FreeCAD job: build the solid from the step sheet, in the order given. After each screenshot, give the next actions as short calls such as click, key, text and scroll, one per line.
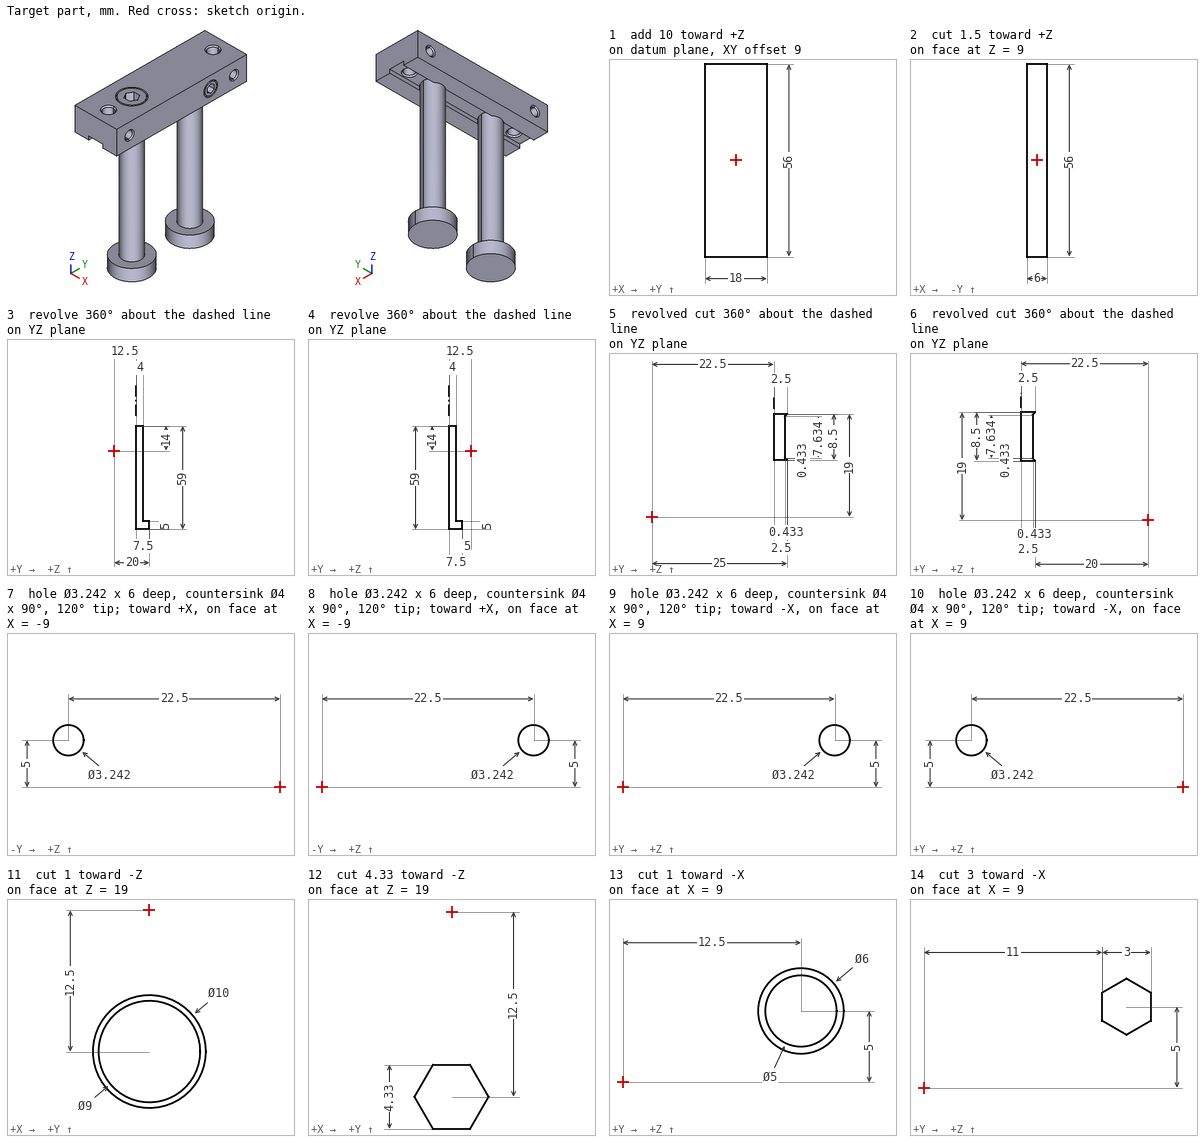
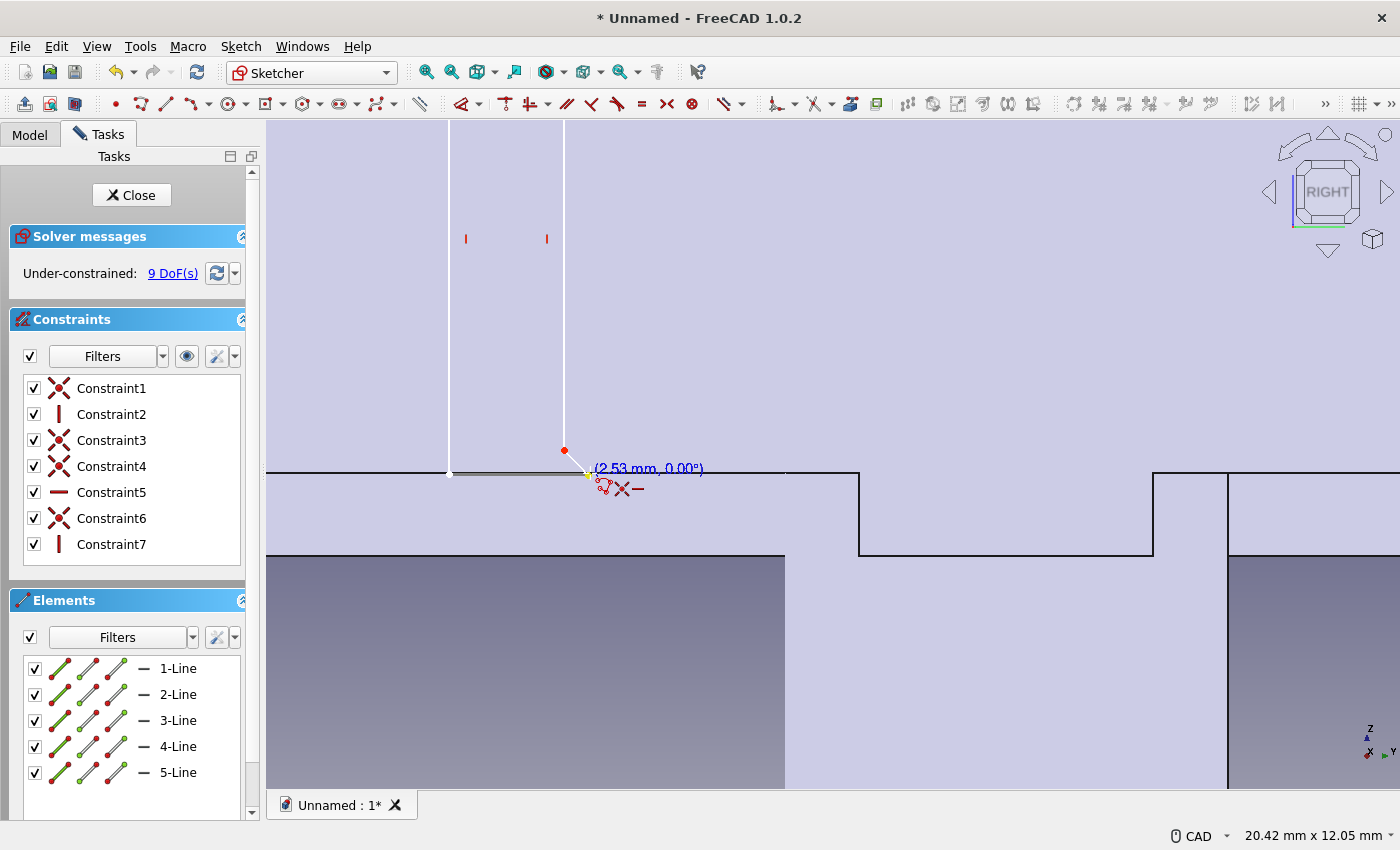
click(588, 476)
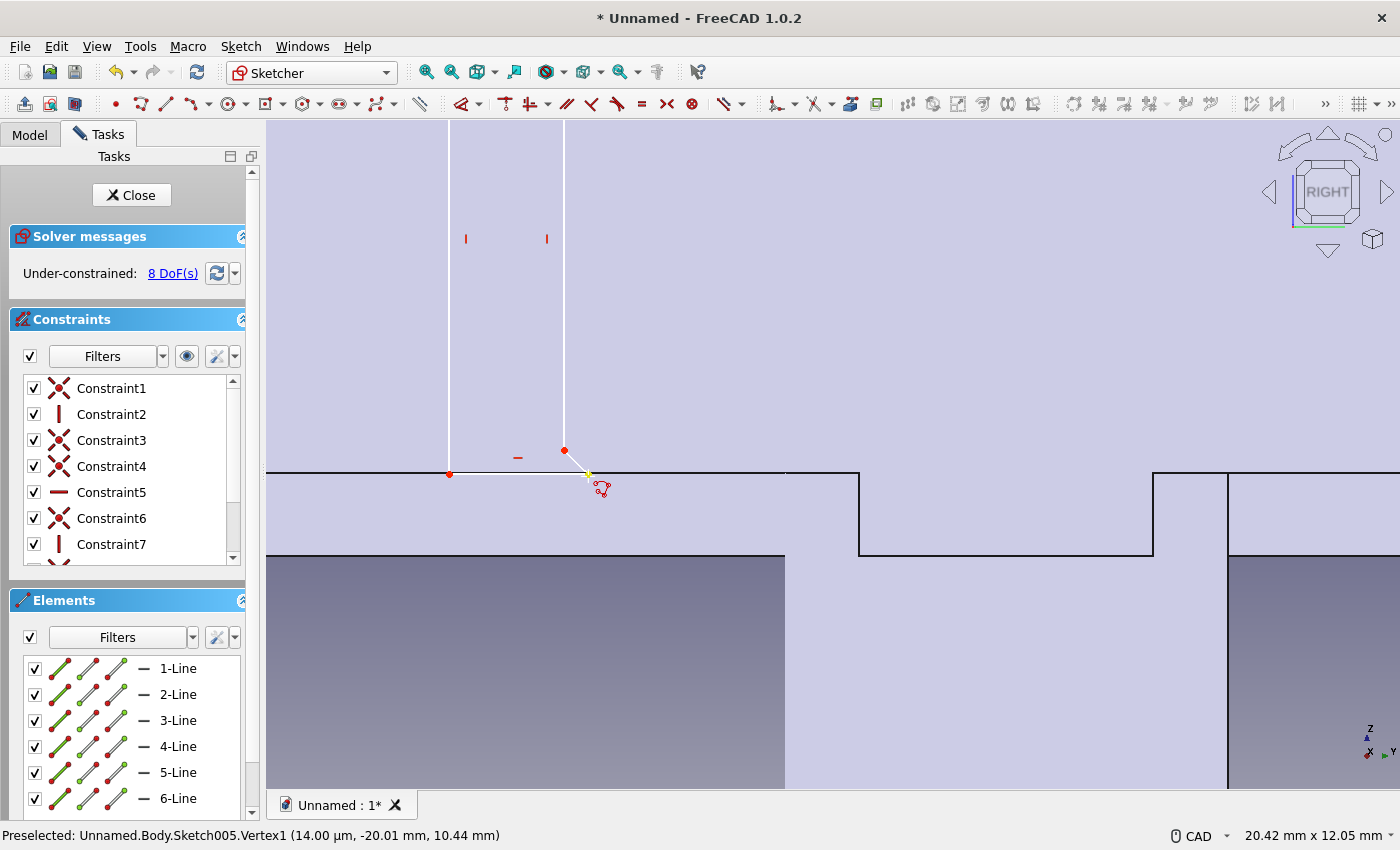
click(166, 104)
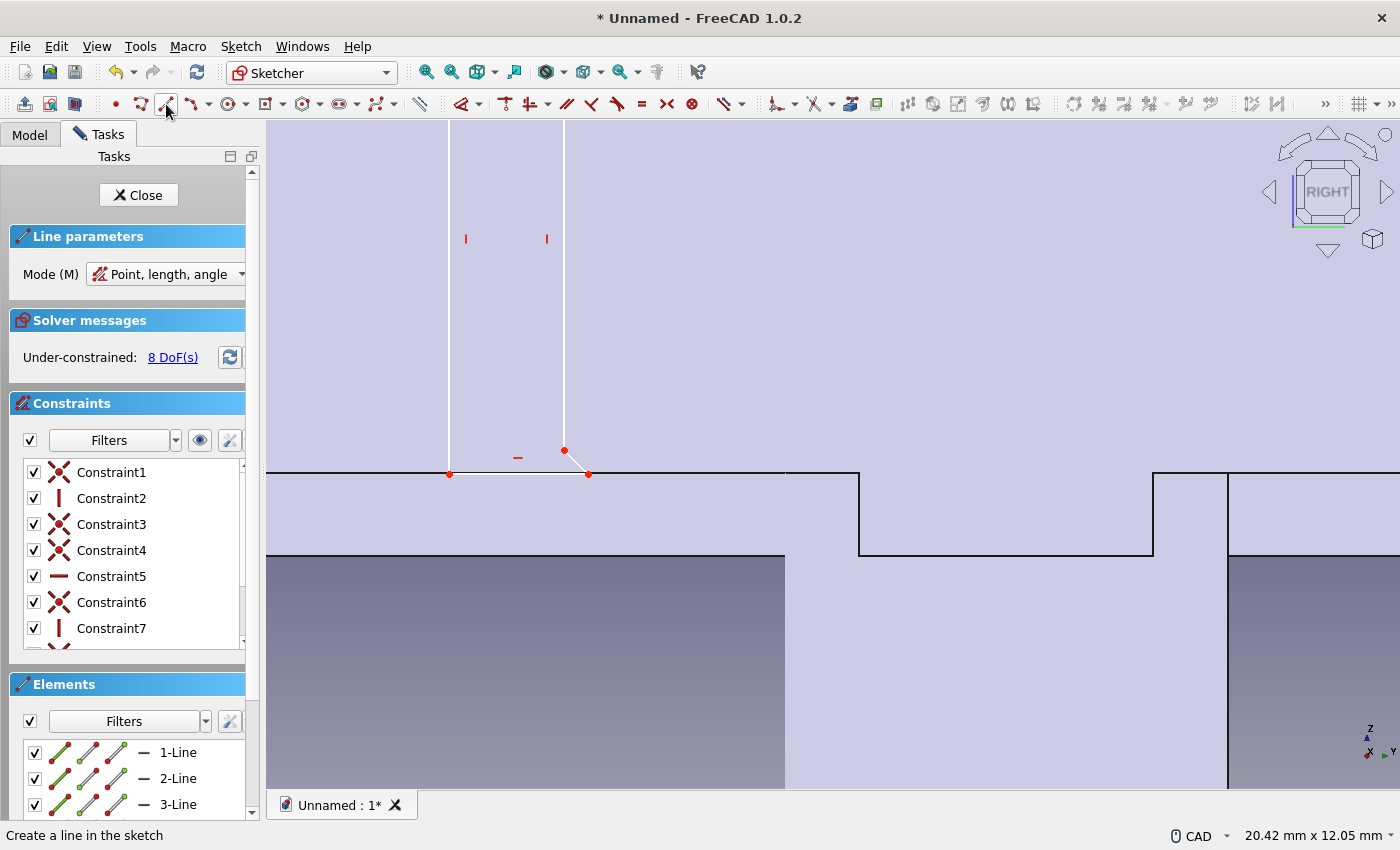
scroll(584, 467, down, 5)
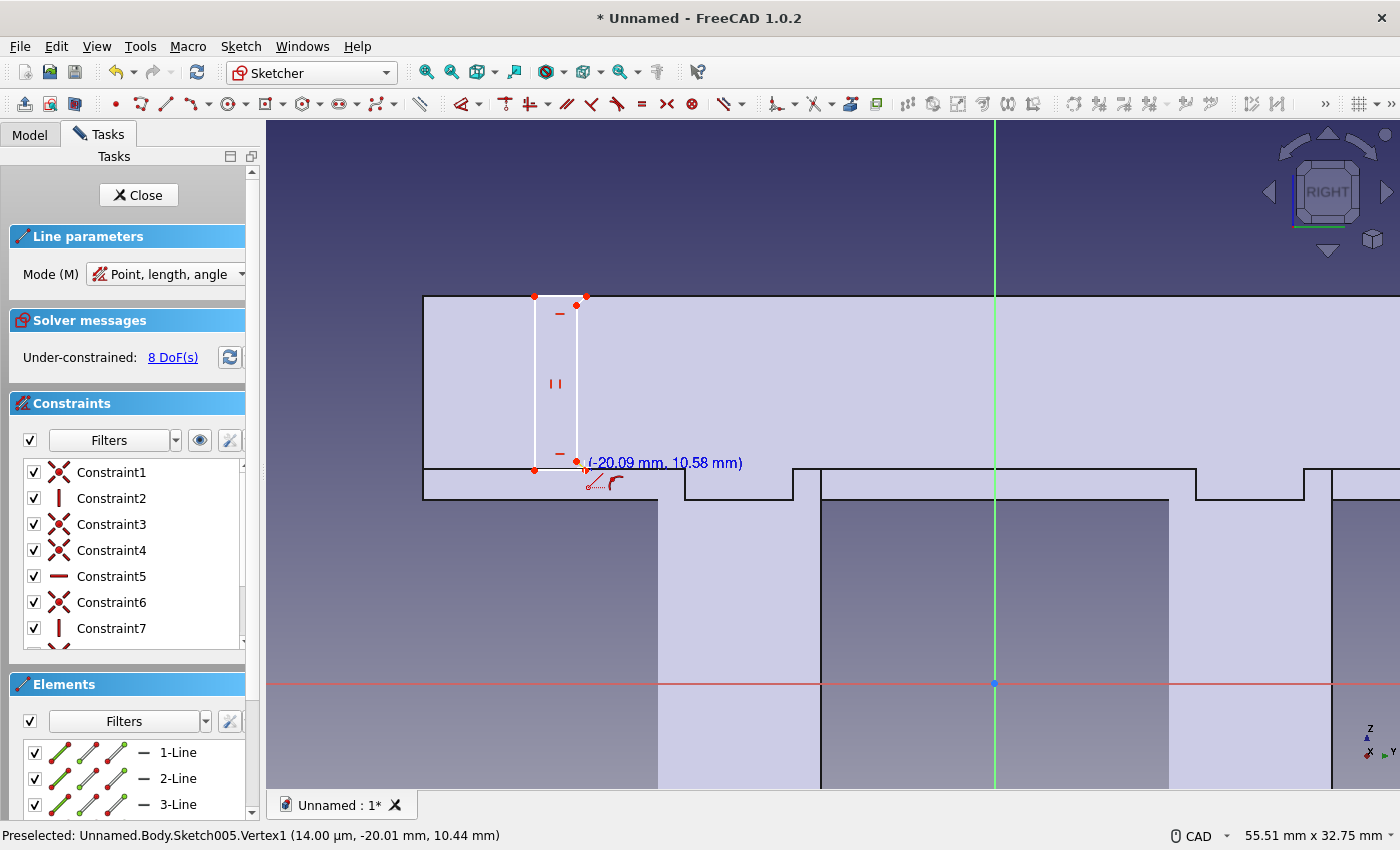
click(535, 278)
click(535, 226)
key(Escape)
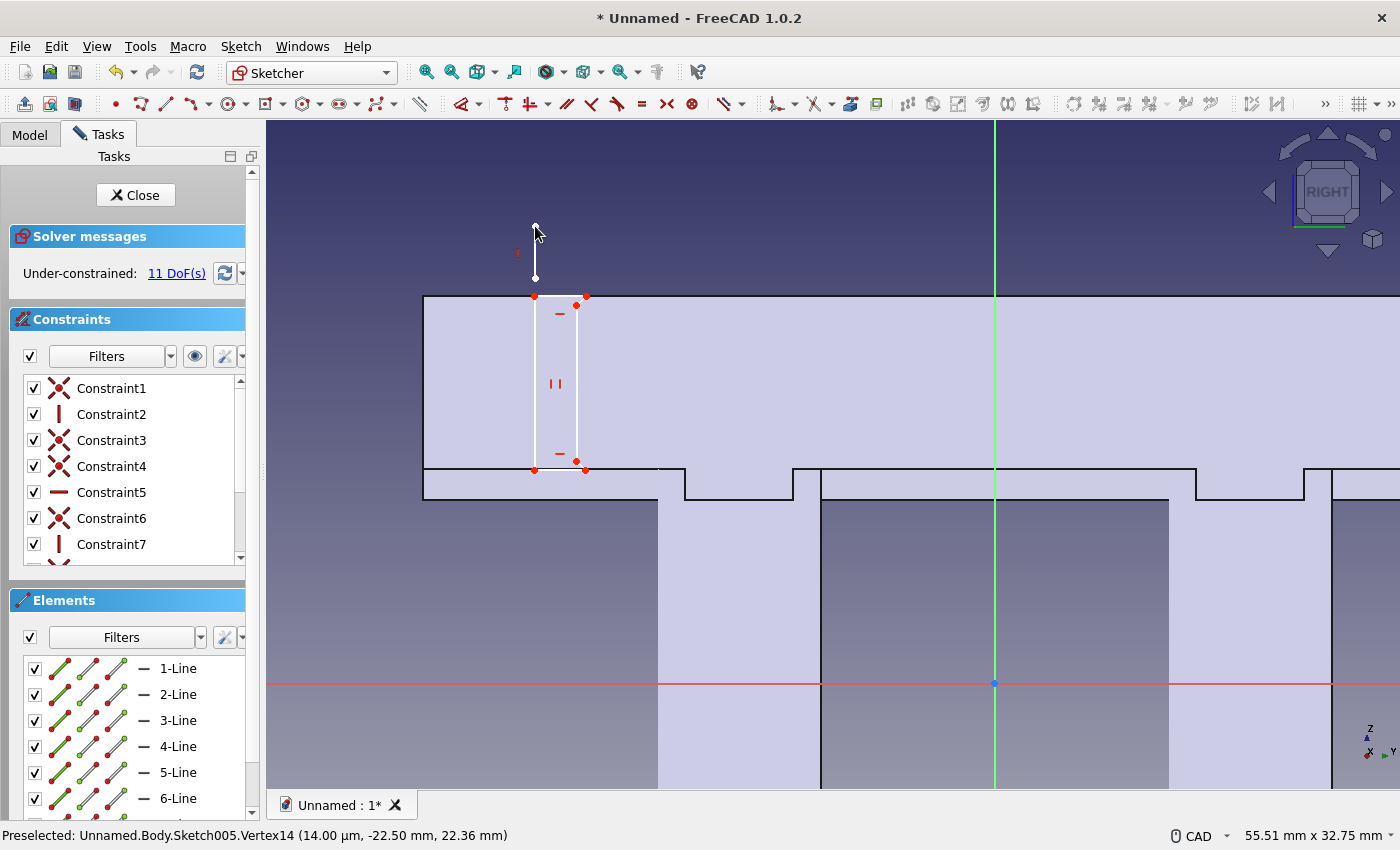
click(535, 263)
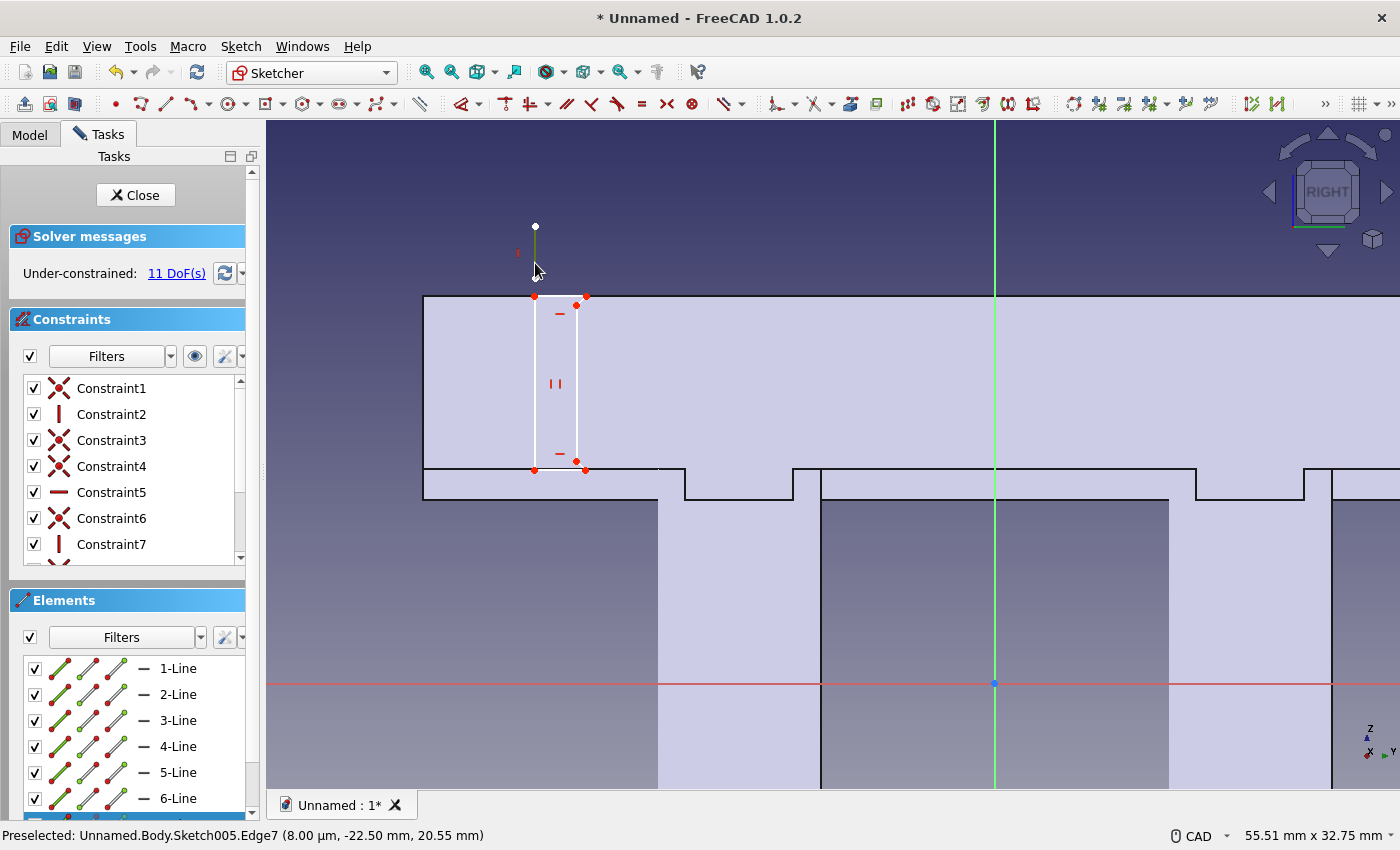
click(420, 104)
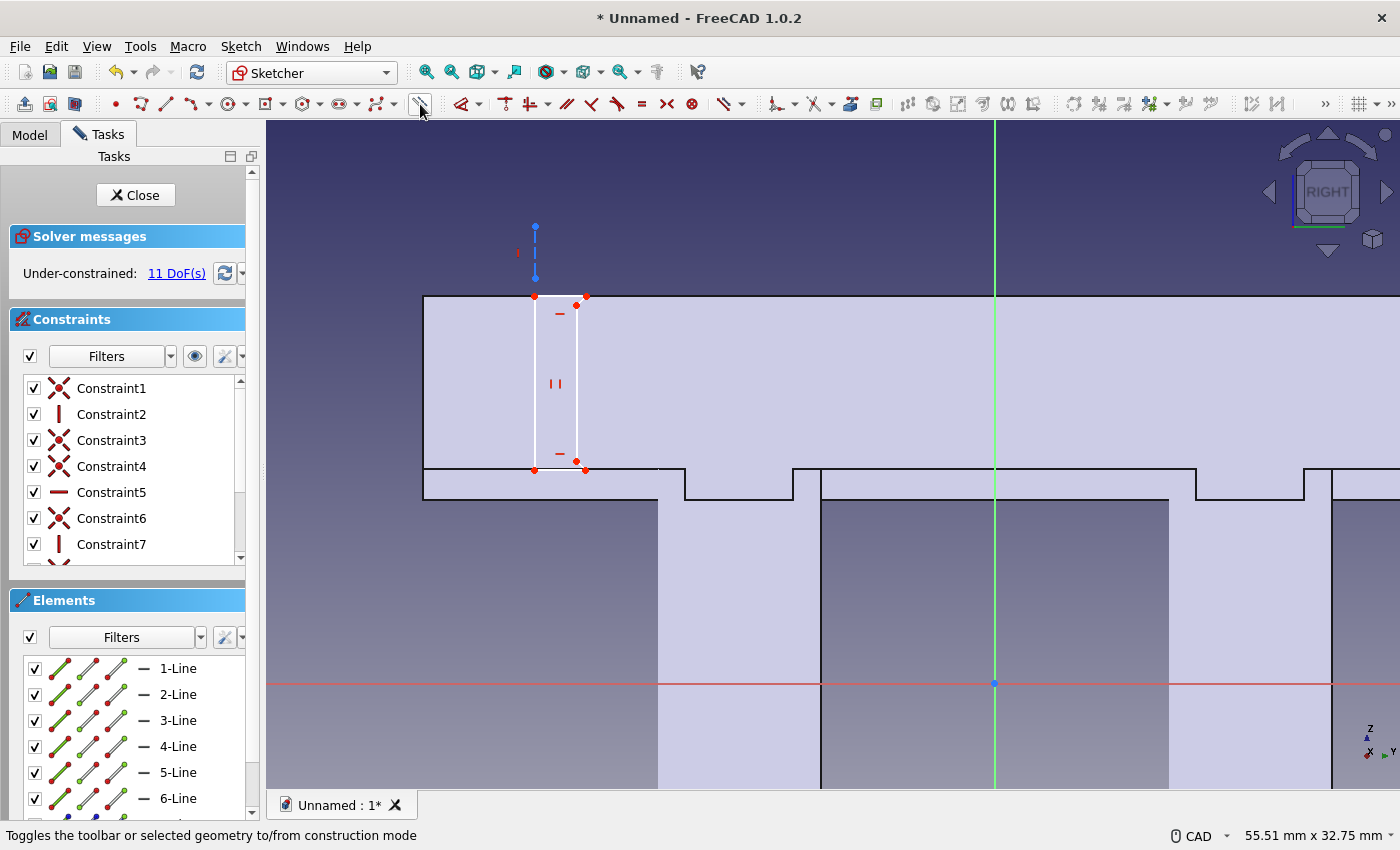
click(460, 104)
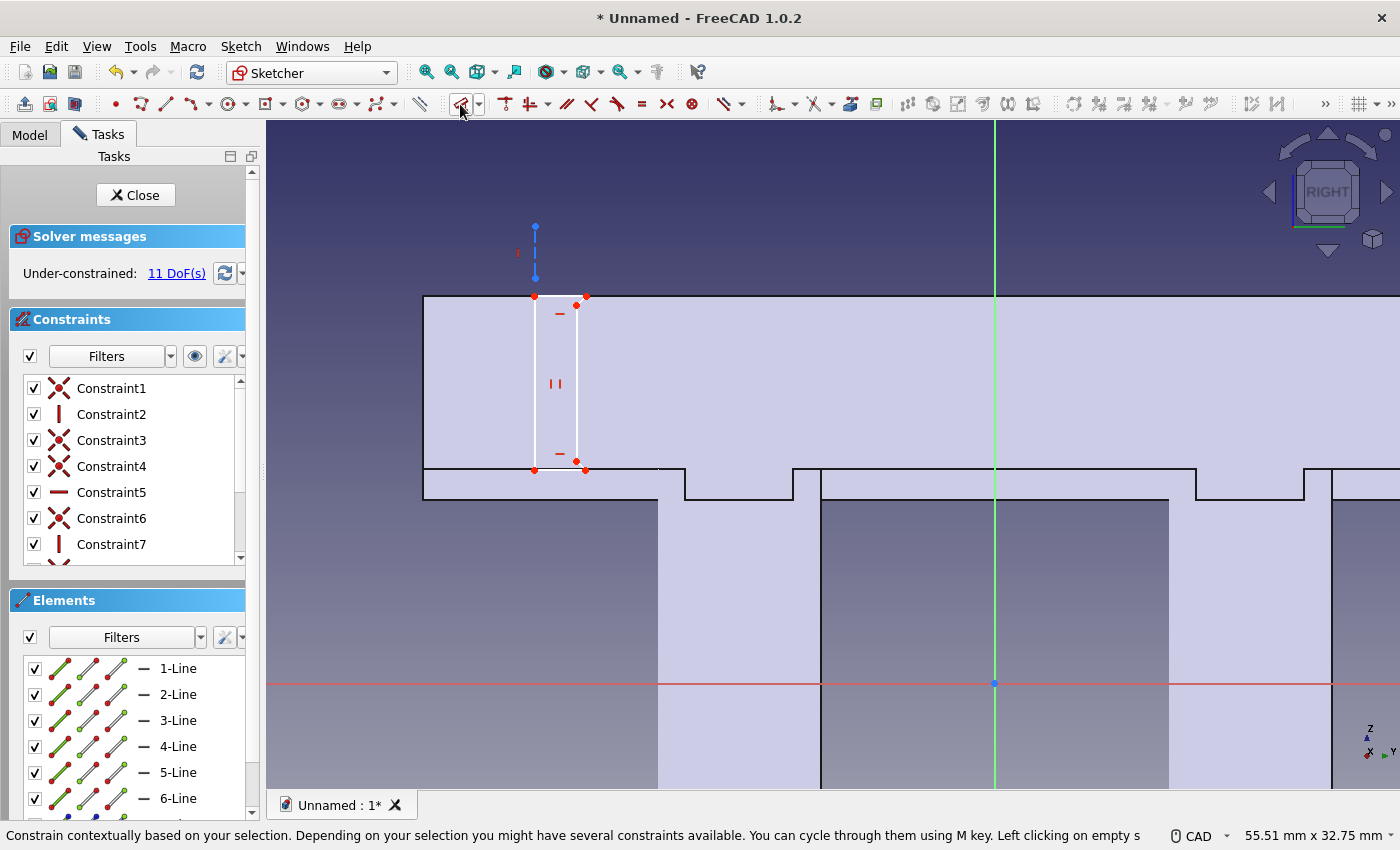
scroll(571, 296, up, 2)